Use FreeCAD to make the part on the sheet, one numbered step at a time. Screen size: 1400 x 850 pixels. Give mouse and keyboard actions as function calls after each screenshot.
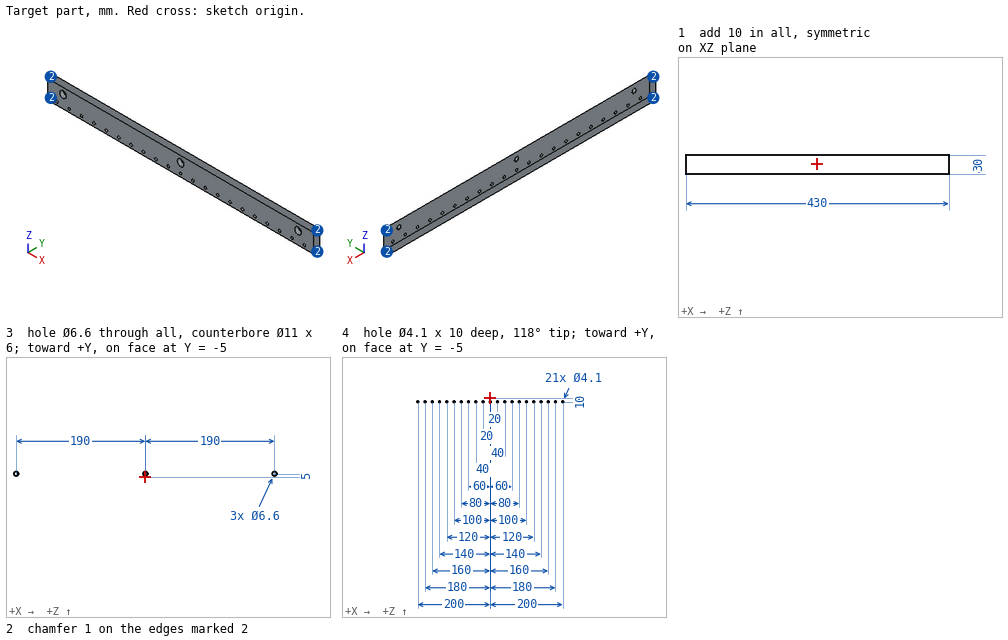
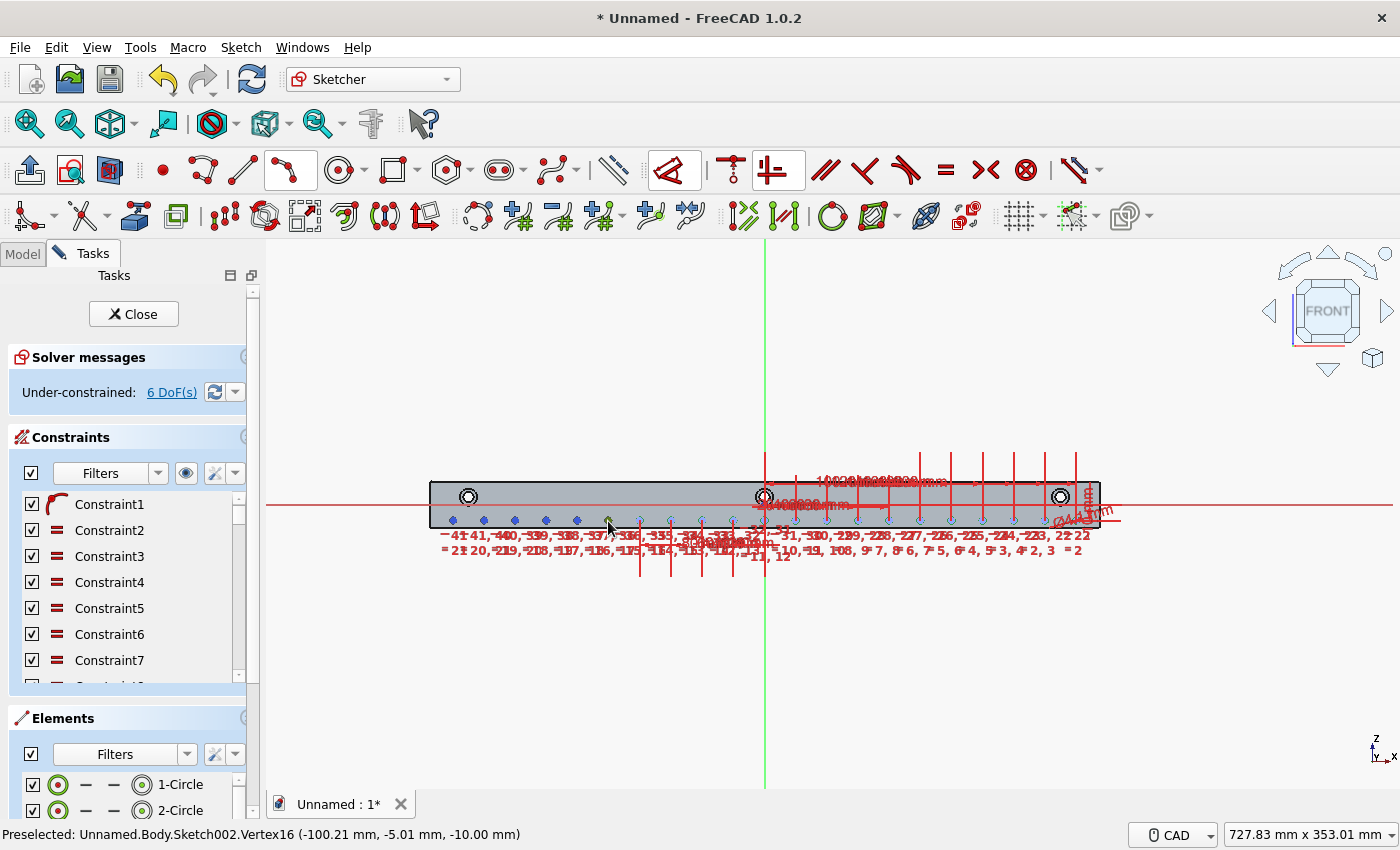
click(696, 170)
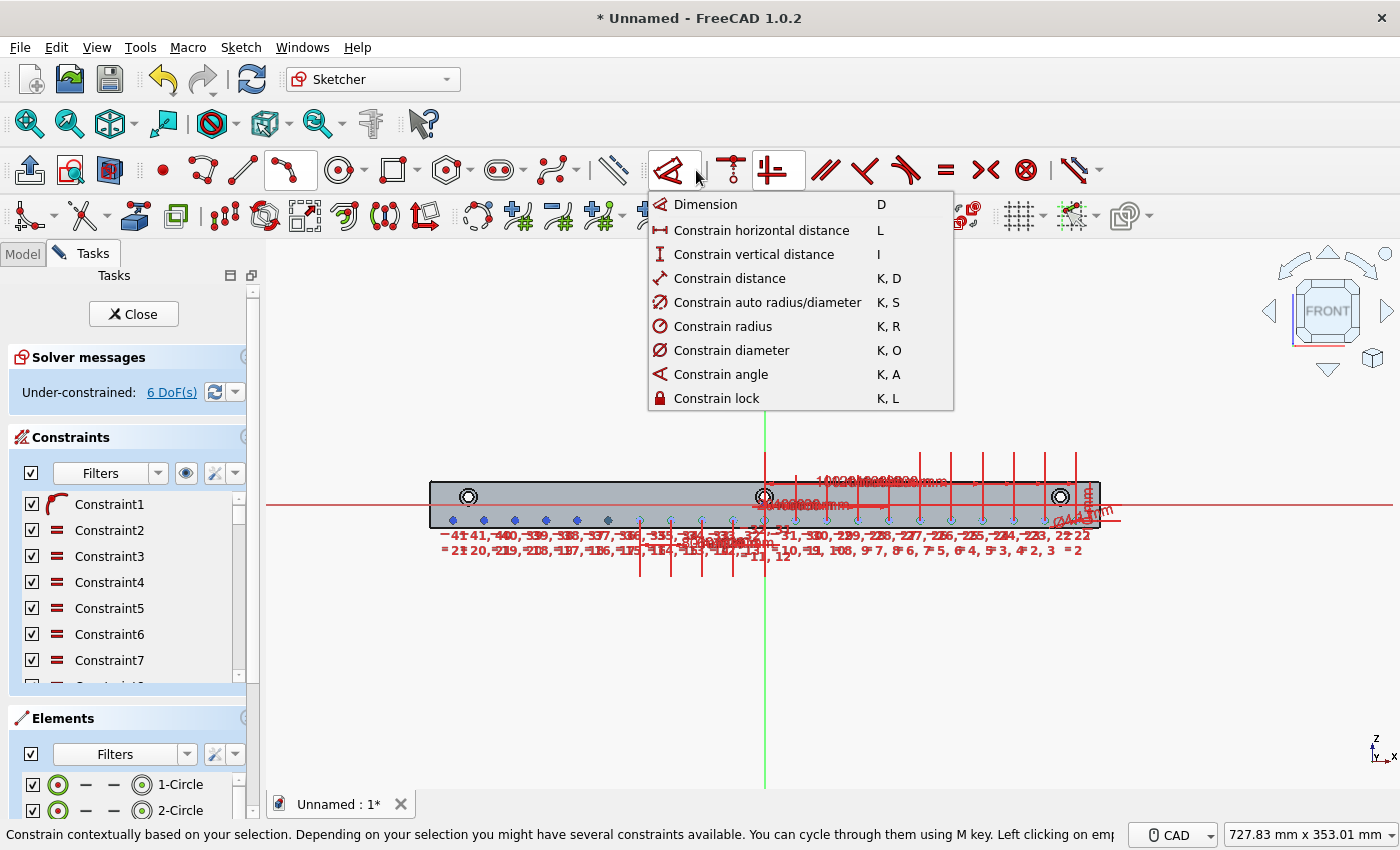
click(801, 230)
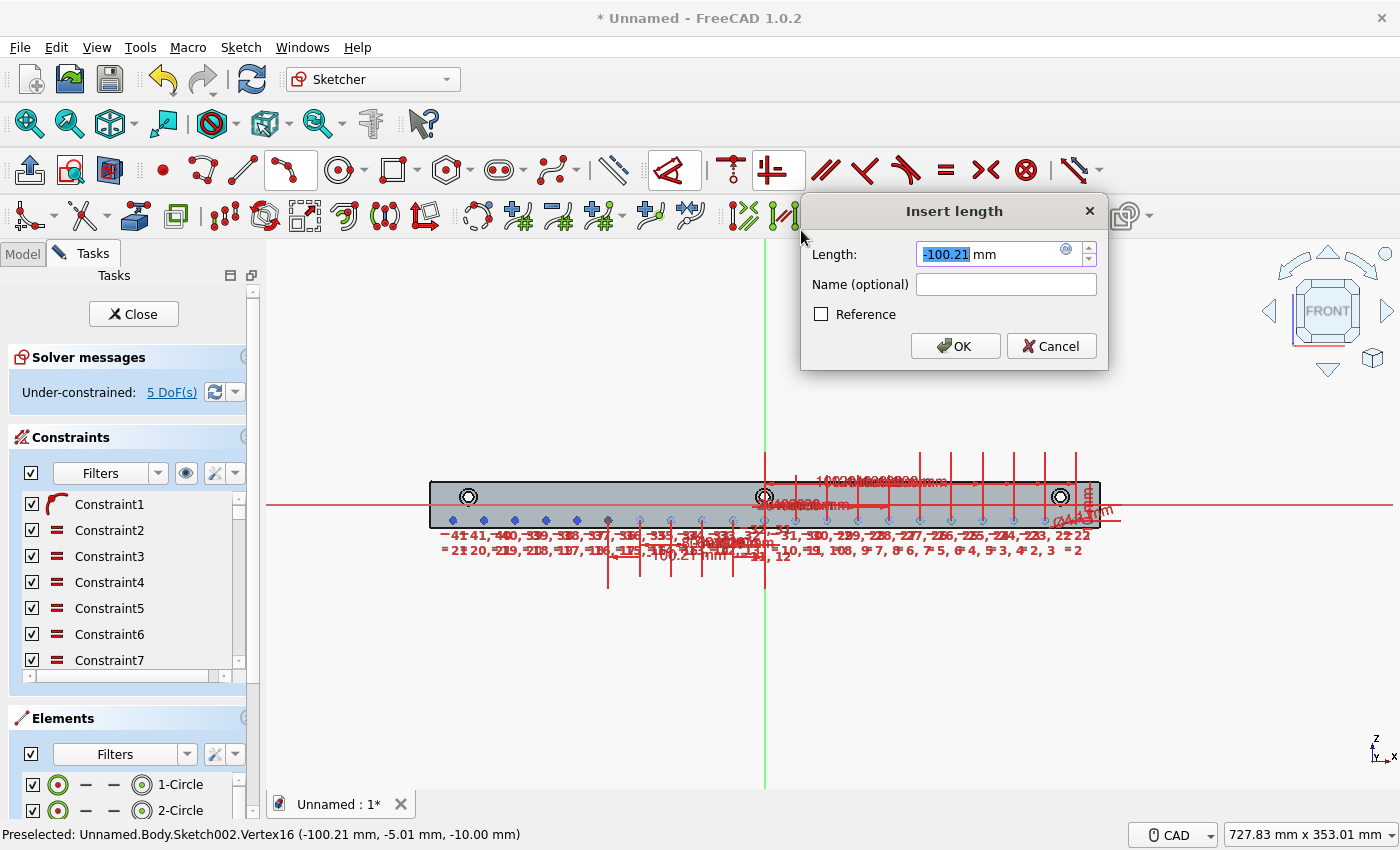
text(-100)
key(Return)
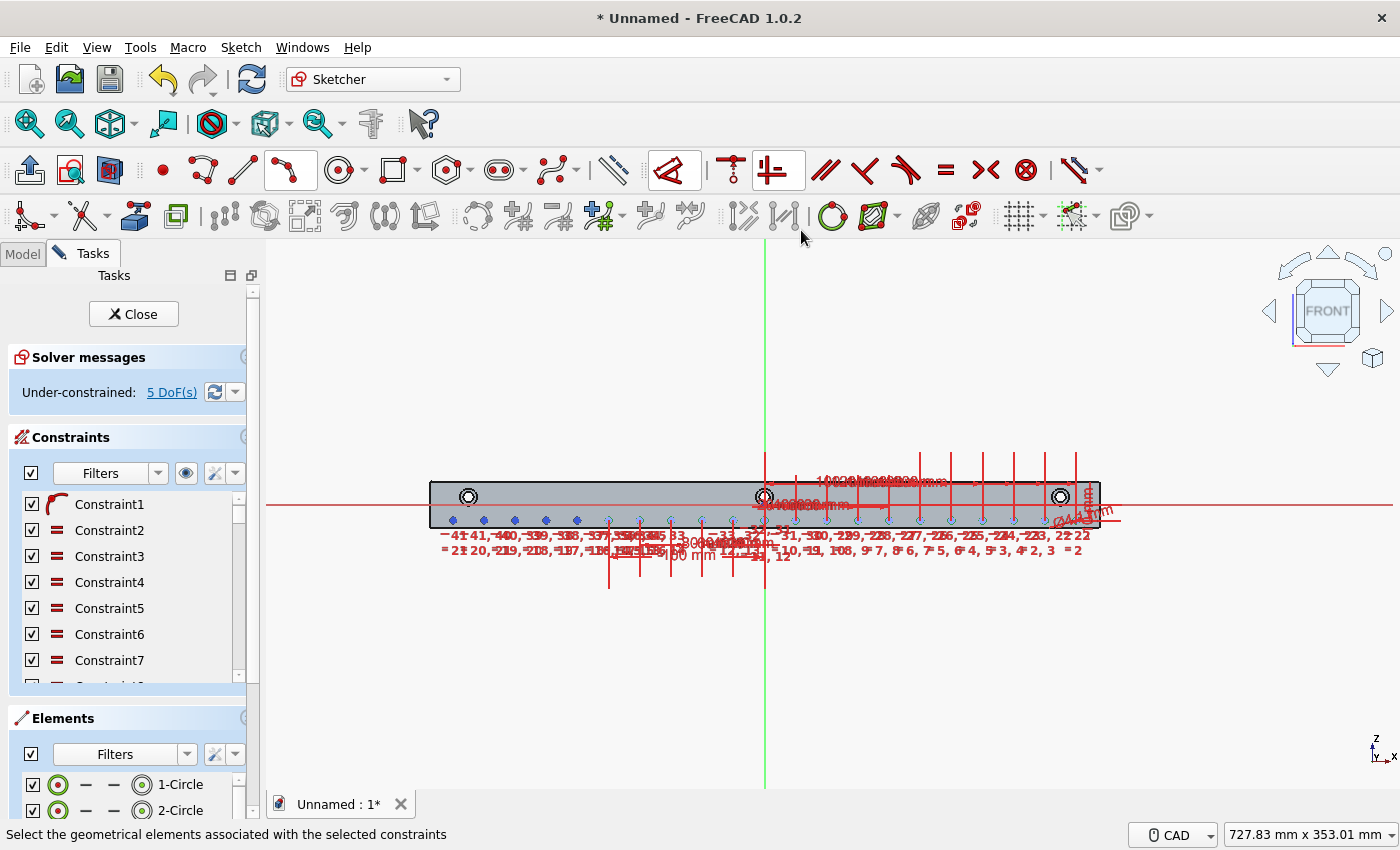
click(577, 521)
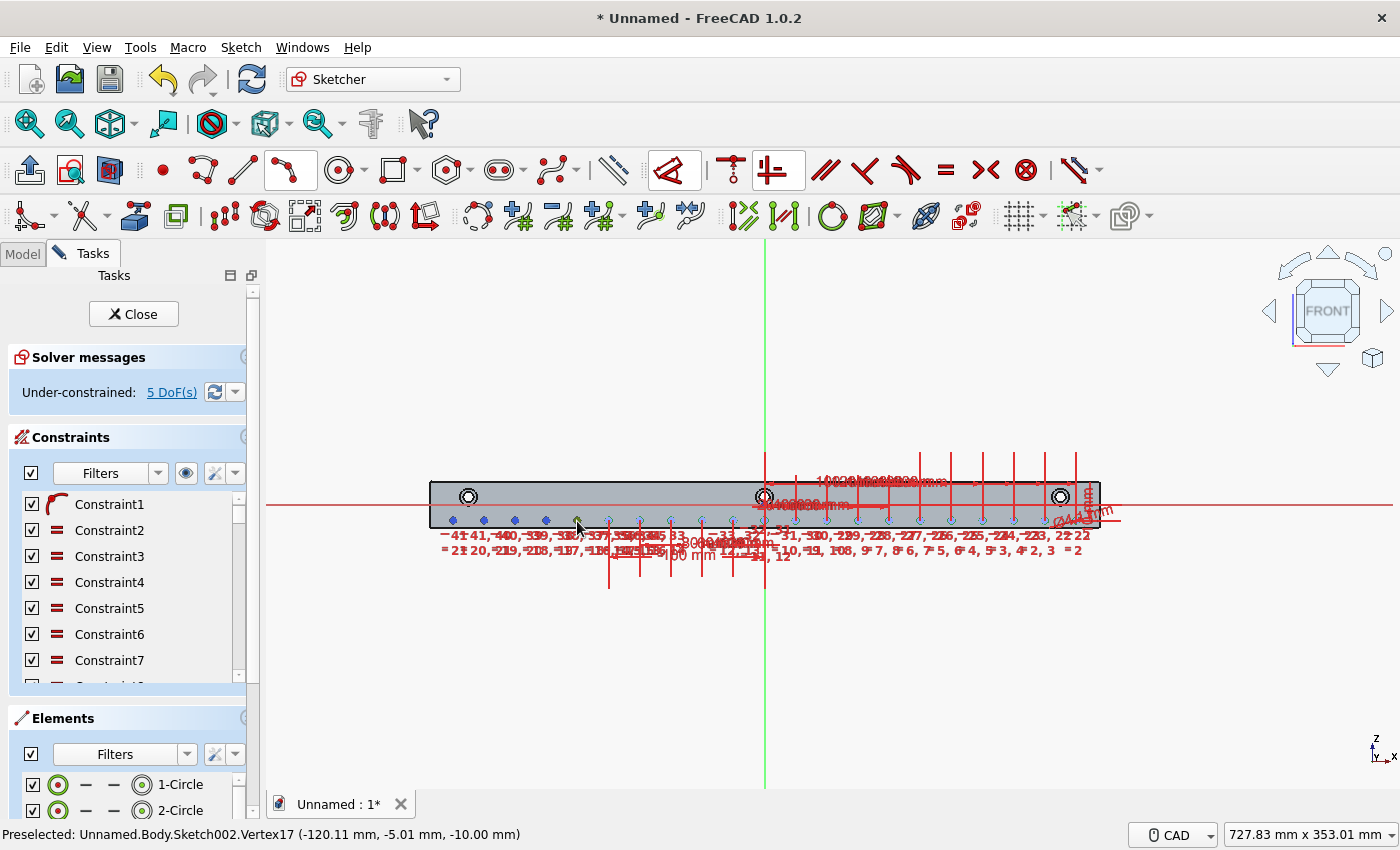
key(l)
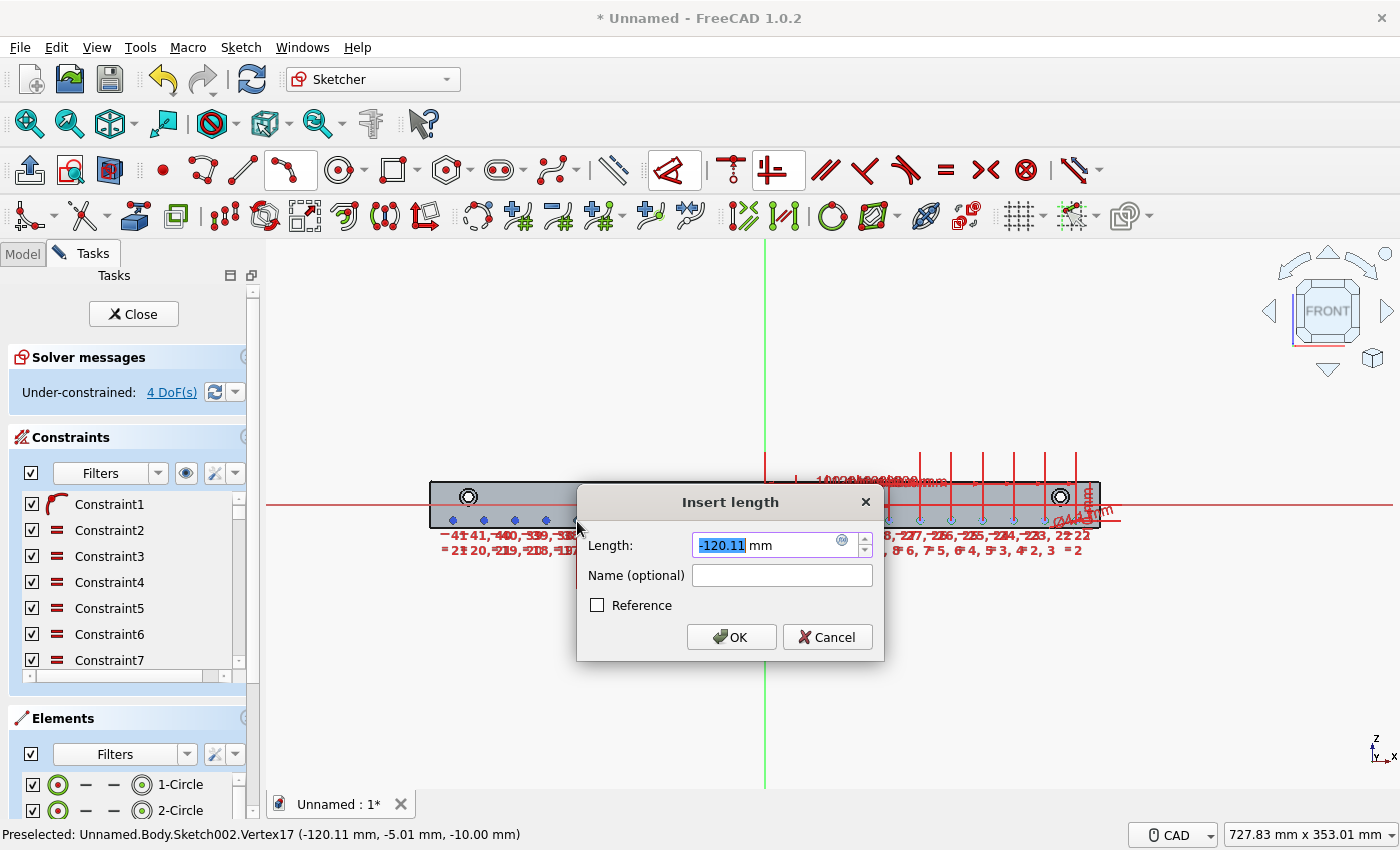
text(-120)
key(Return)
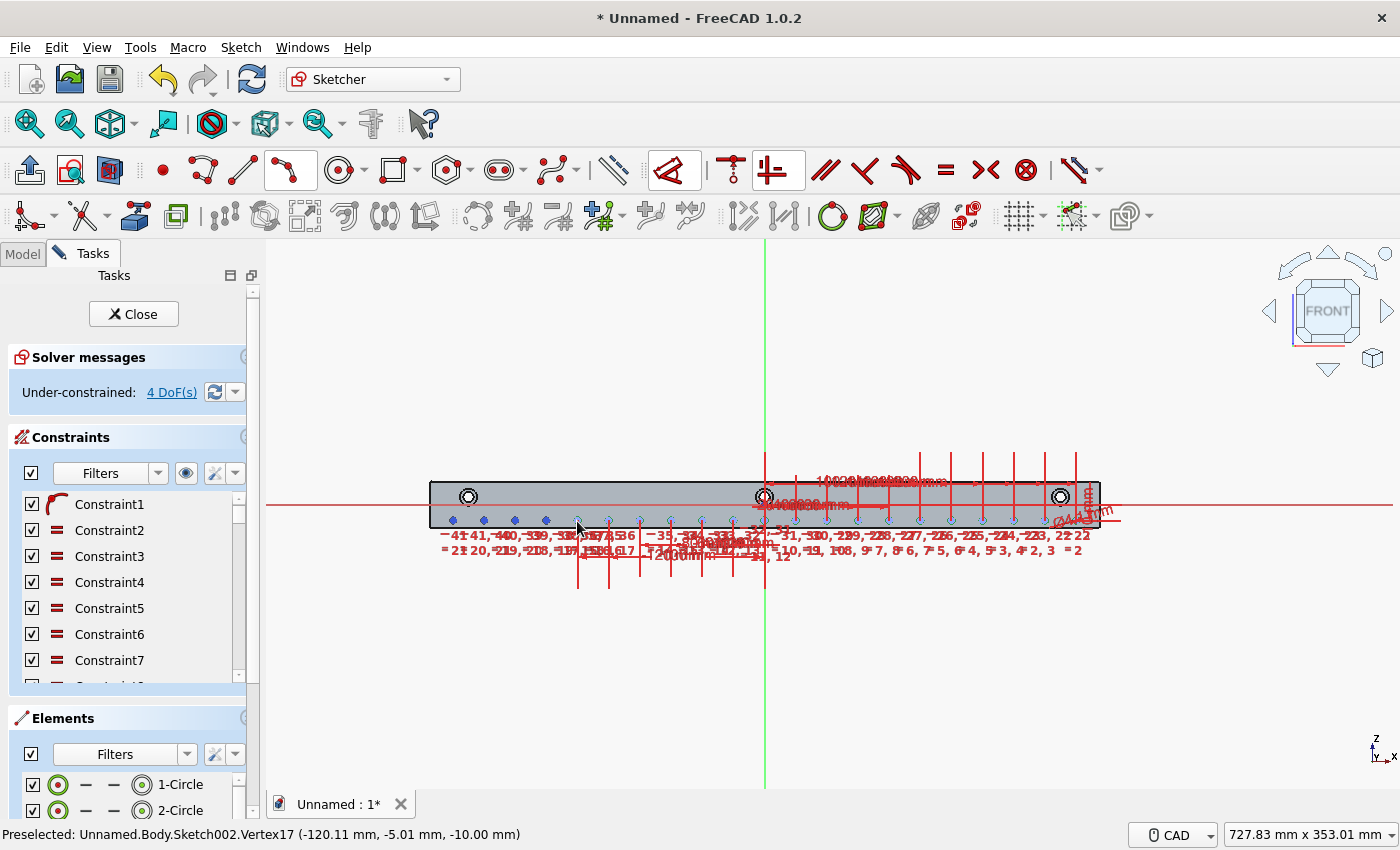
click(546, 521)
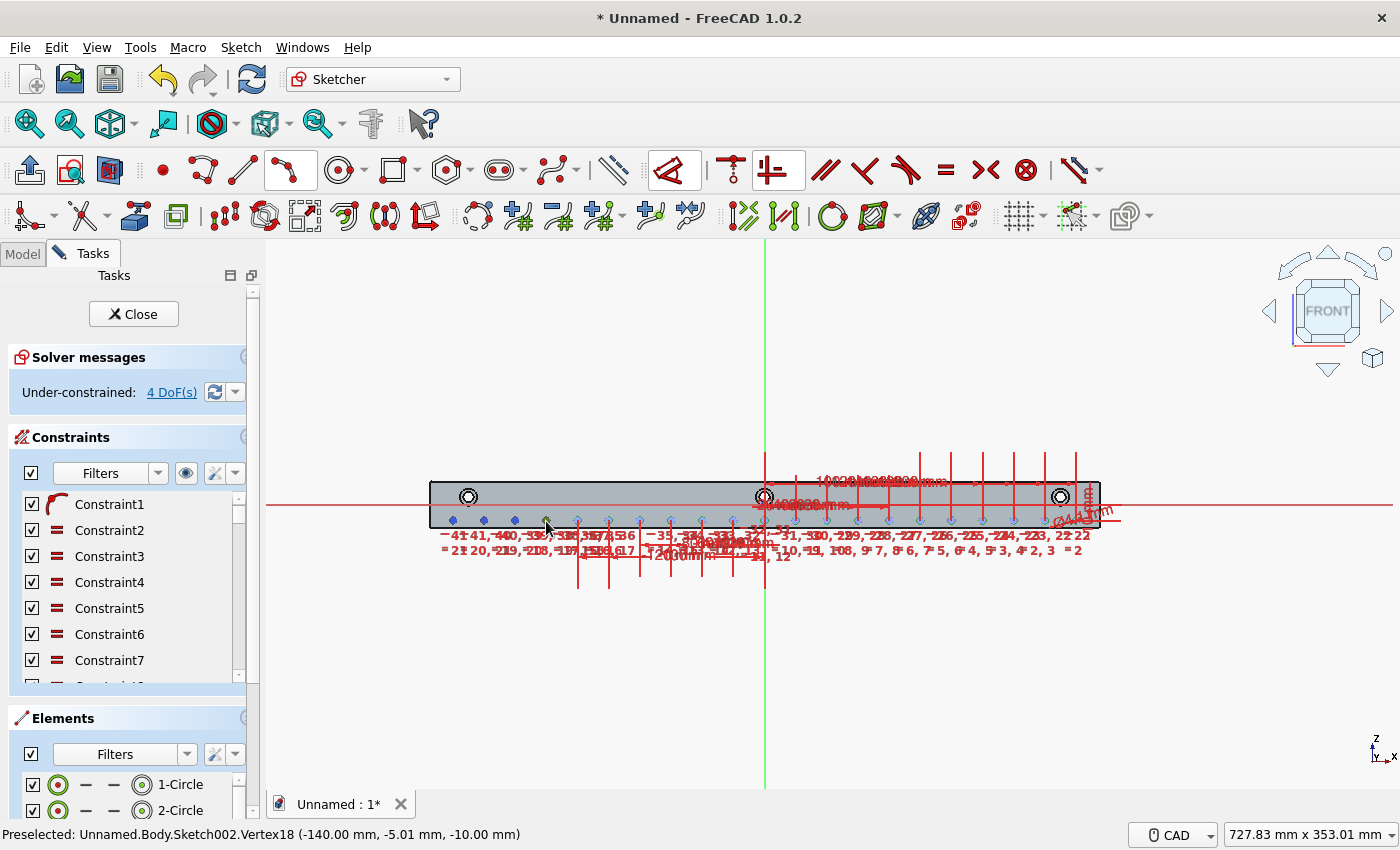
key(l)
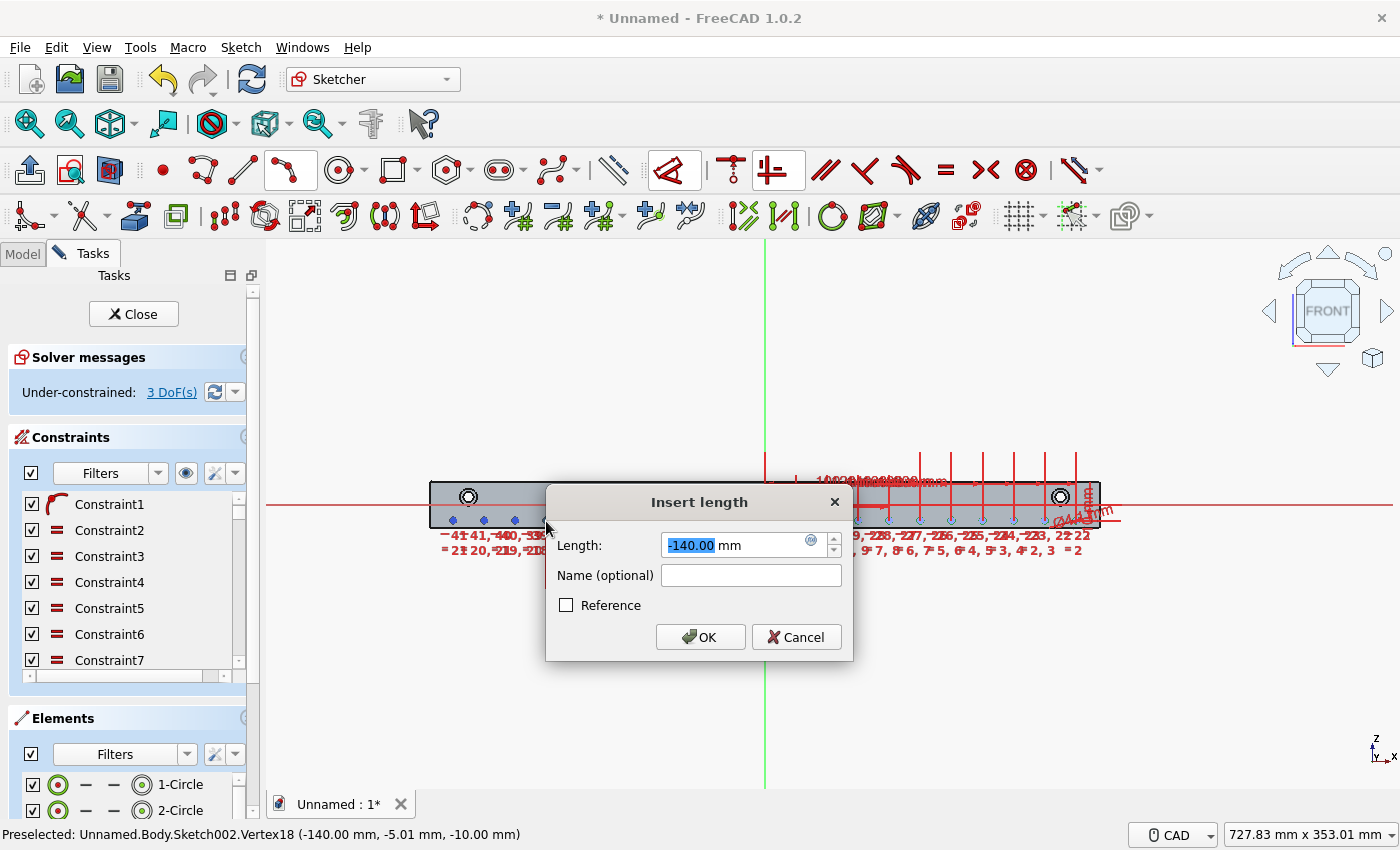
text(-140)
key(Return)